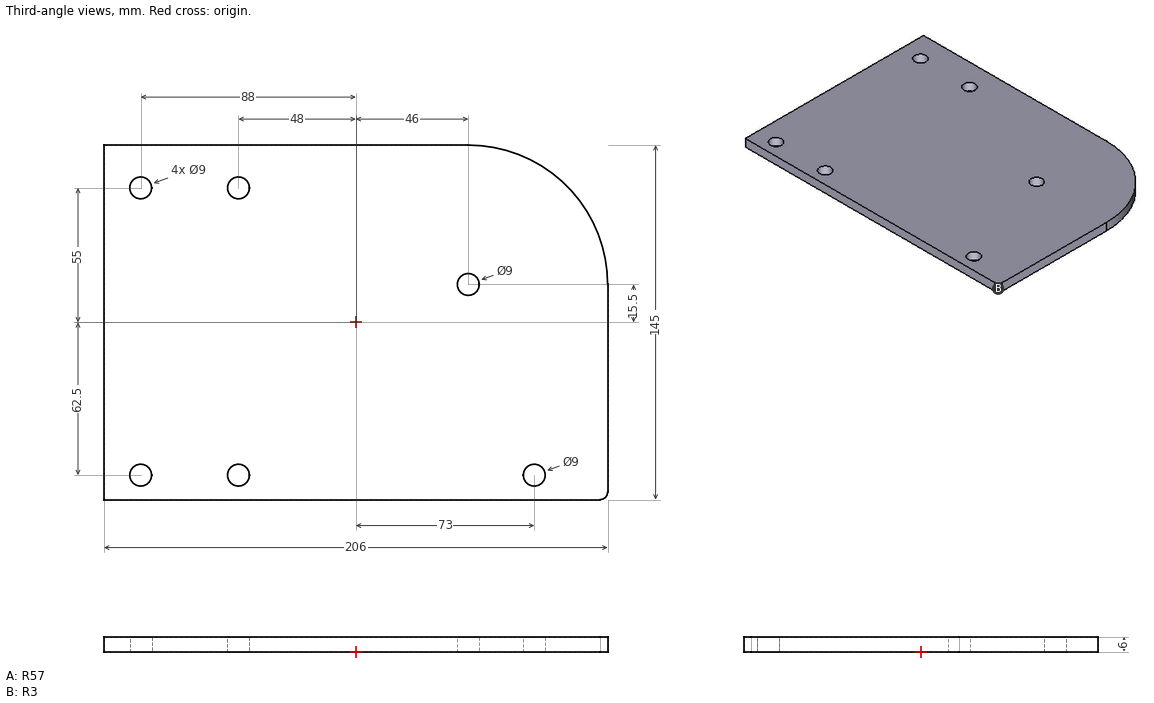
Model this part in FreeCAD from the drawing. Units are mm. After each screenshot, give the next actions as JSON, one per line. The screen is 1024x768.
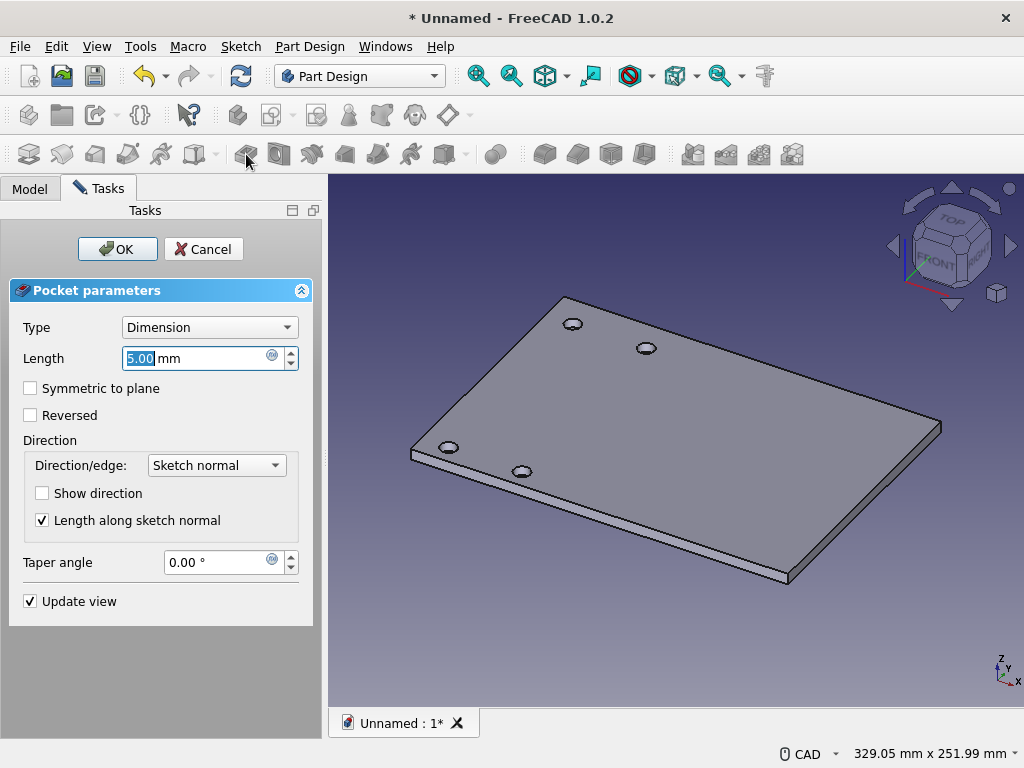
{"action": "left_click", "coordinate": [210, 328]}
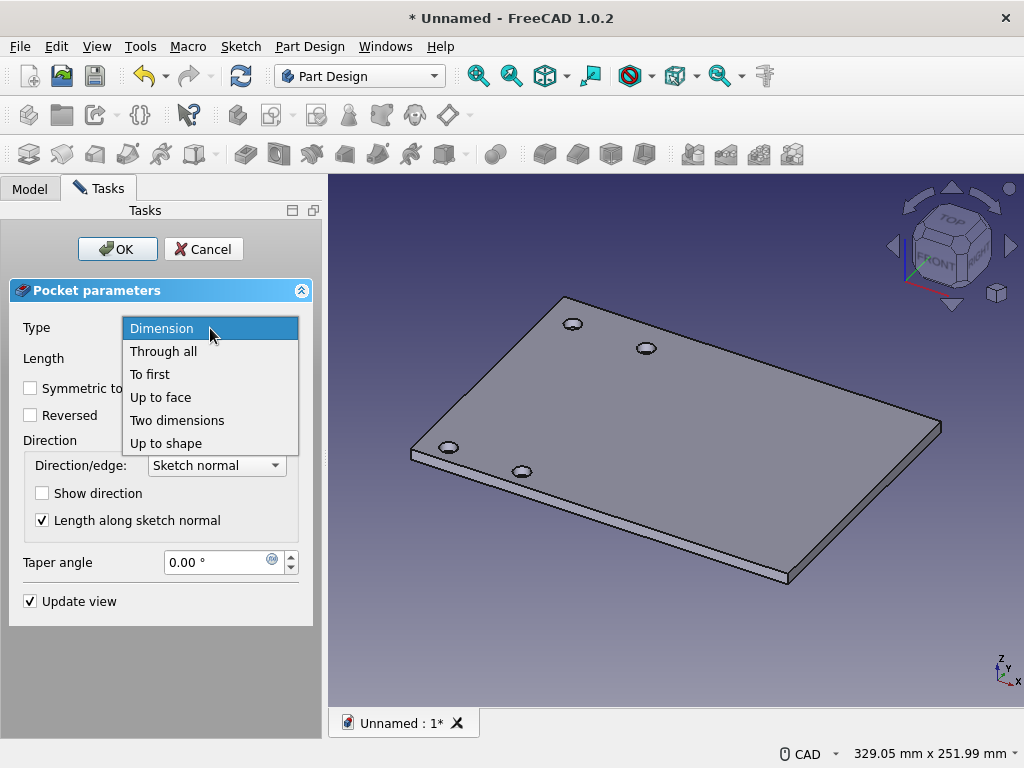
{"action": "left_click", "coordinate": [208, 352]}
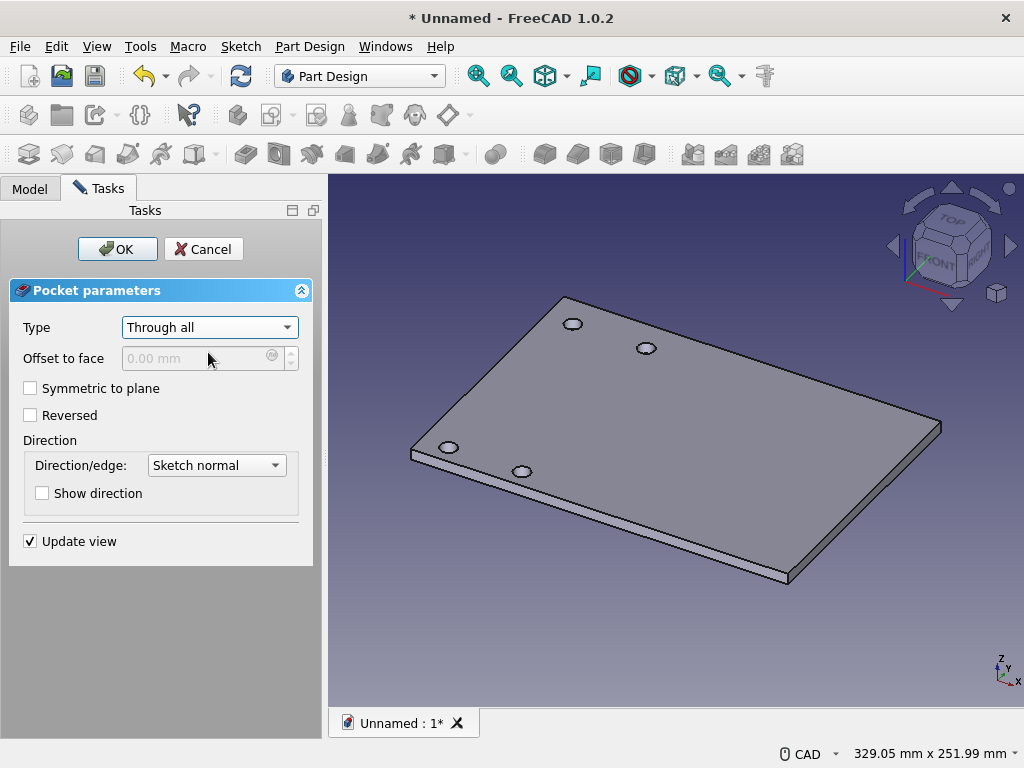
{"action": "left_click", "coordinate": [118, 249]}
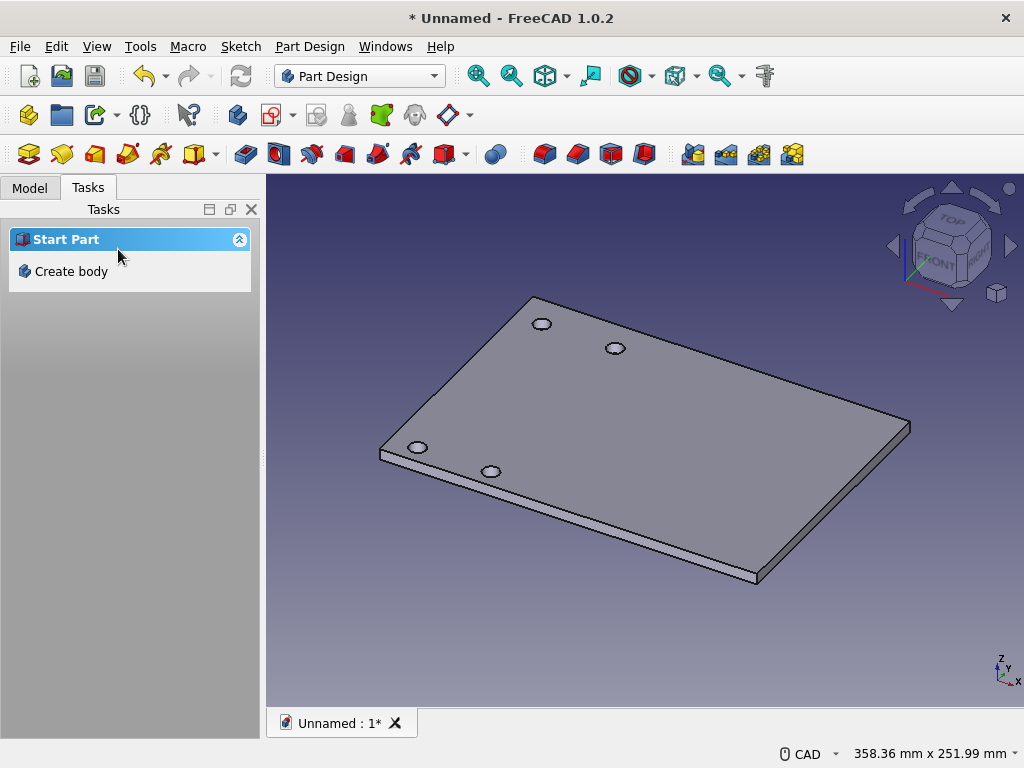
{"action": "left_click", "coordinate": [699, 452]}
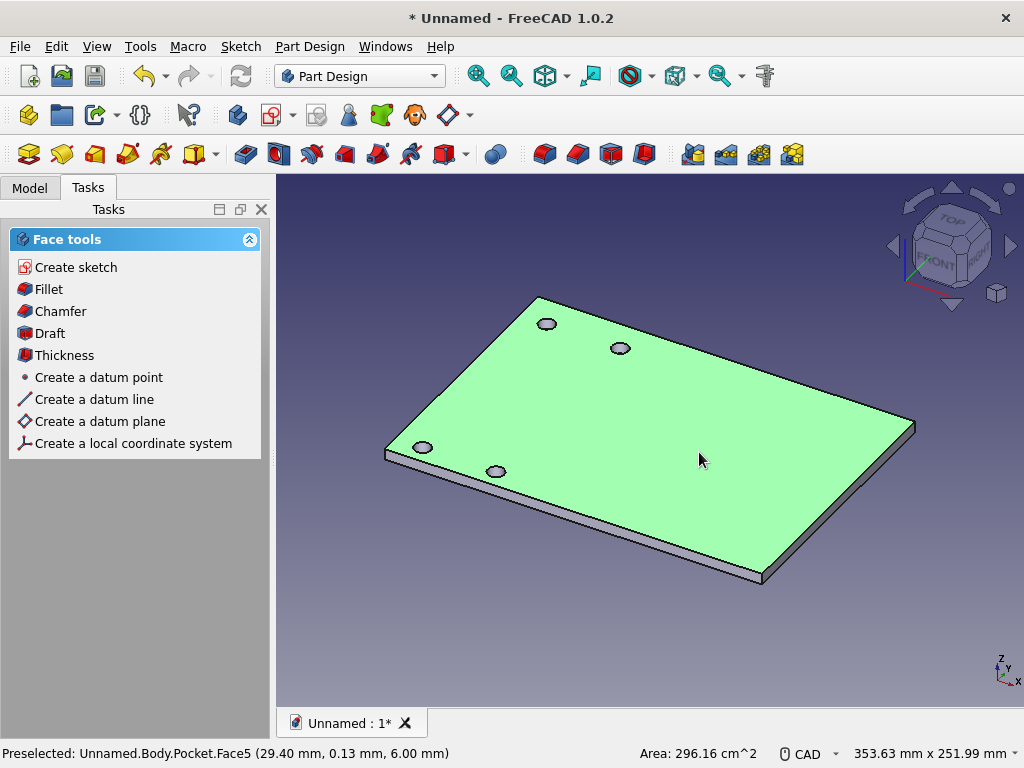
{"action": "left_click", "coordinate": [270, 116]}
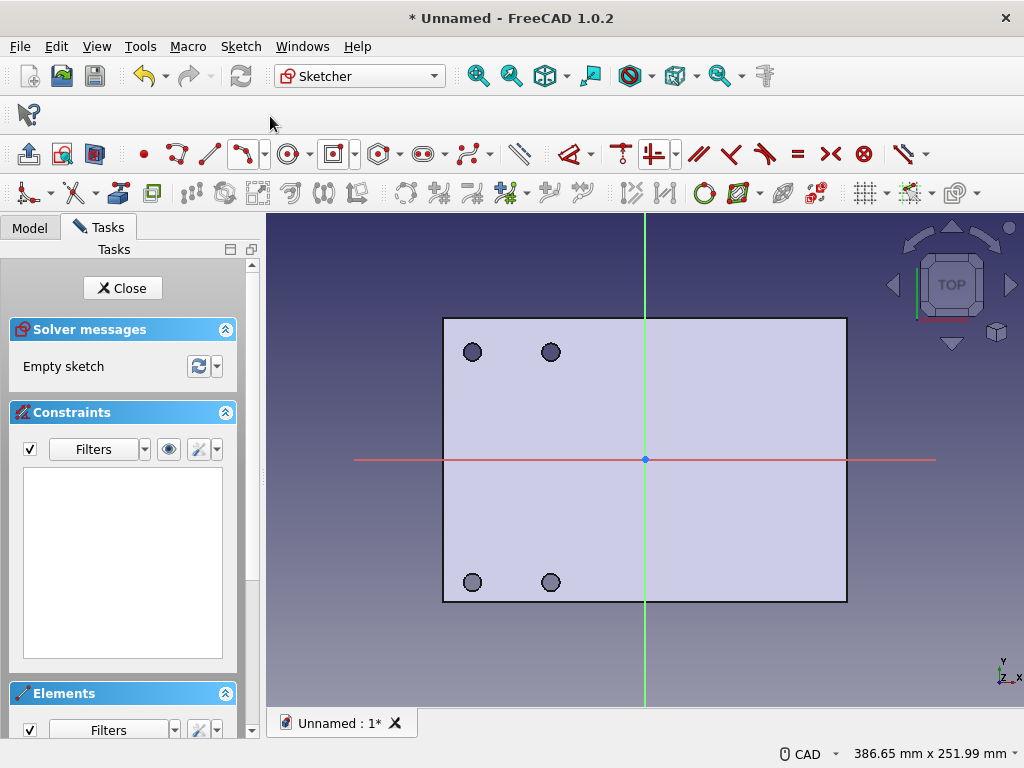
{"action": "scroll", "coordinate": [745, 428], "scroll_direction": "up", "scroll_amount": 14}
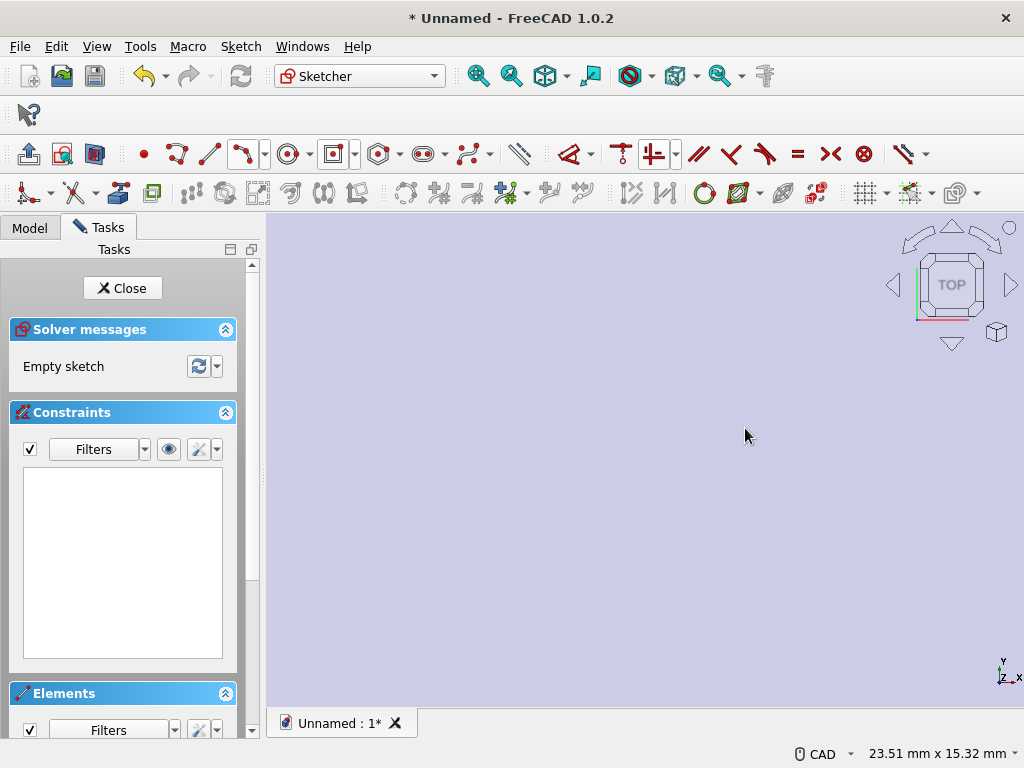
{"action": "key", "text": "g c"}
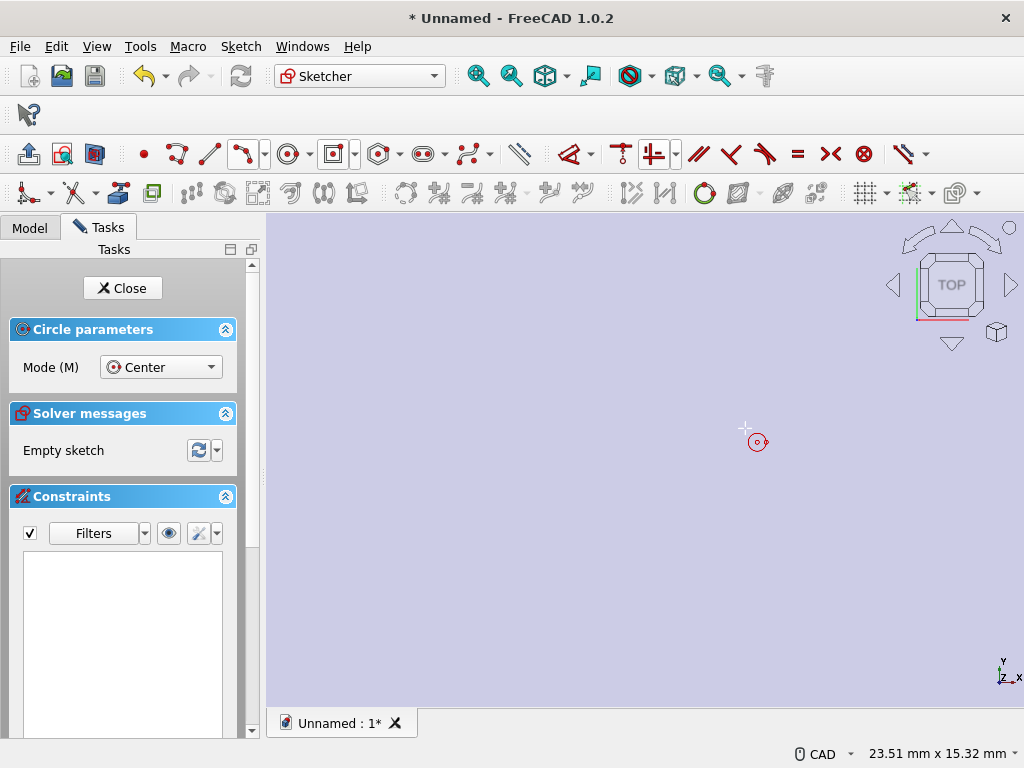
{"action": "left_click", "coordinate": [574, 448]}
{"action": "mouse_move", "coordinate": [676, 345]}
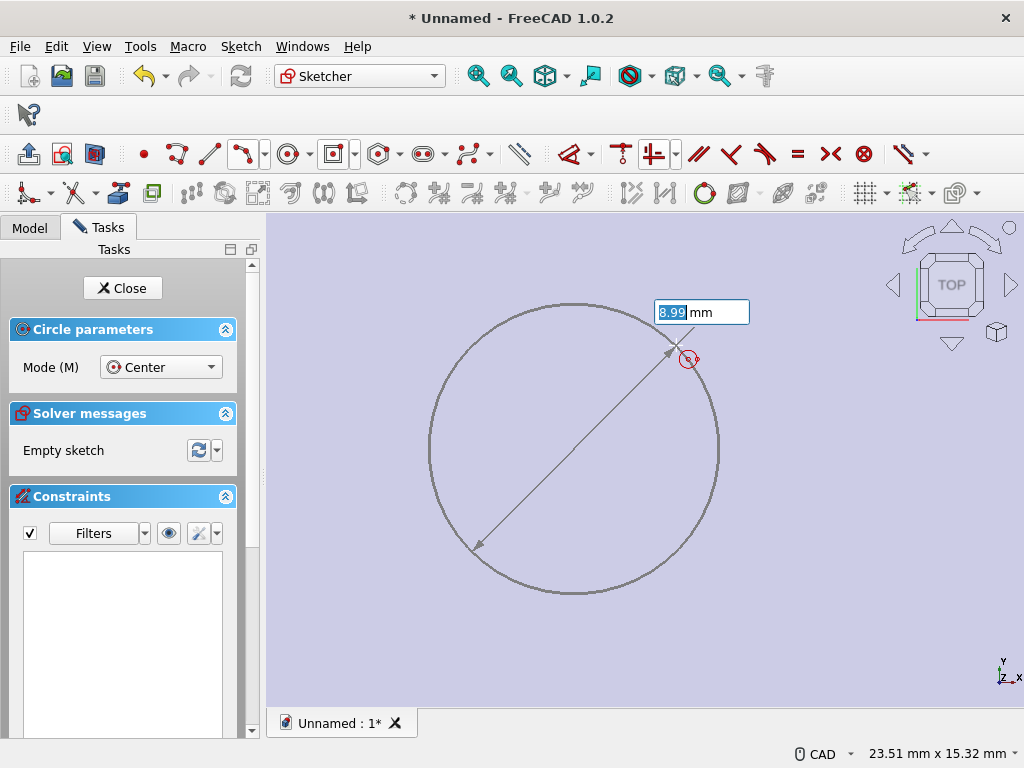
{"action": "type", "text": "9"}
{"action": "key", "text": "Return"}
{"action": "key", "text": "Escape"}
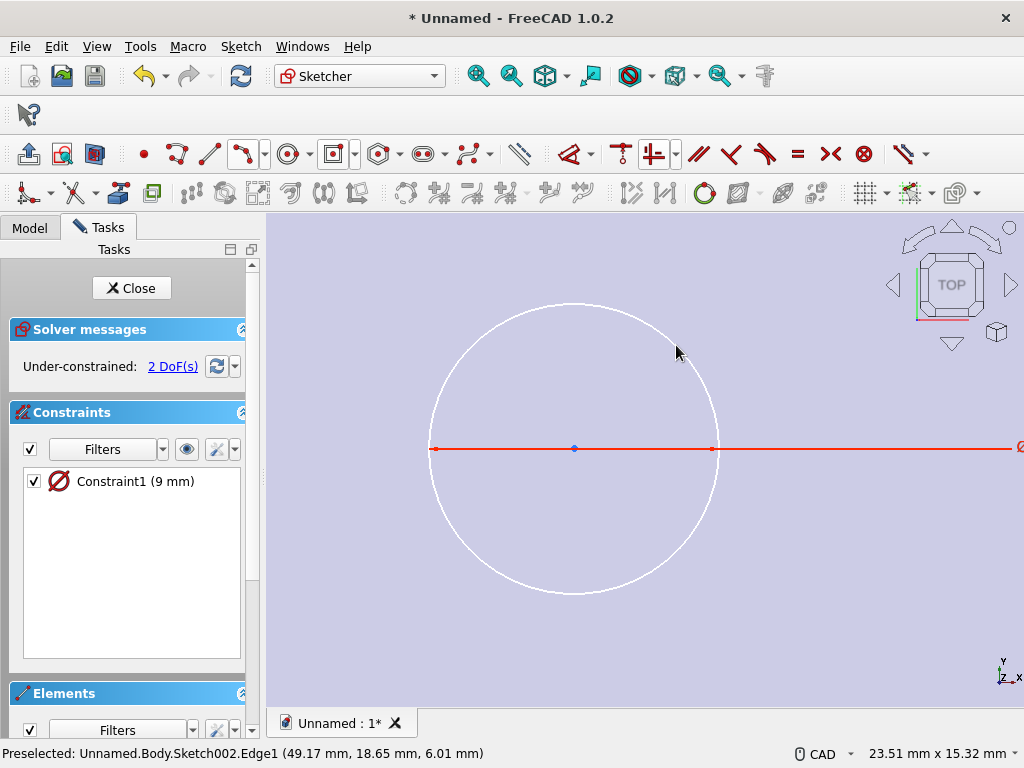
{"action": "left_click", "coordinate": [568, 154]}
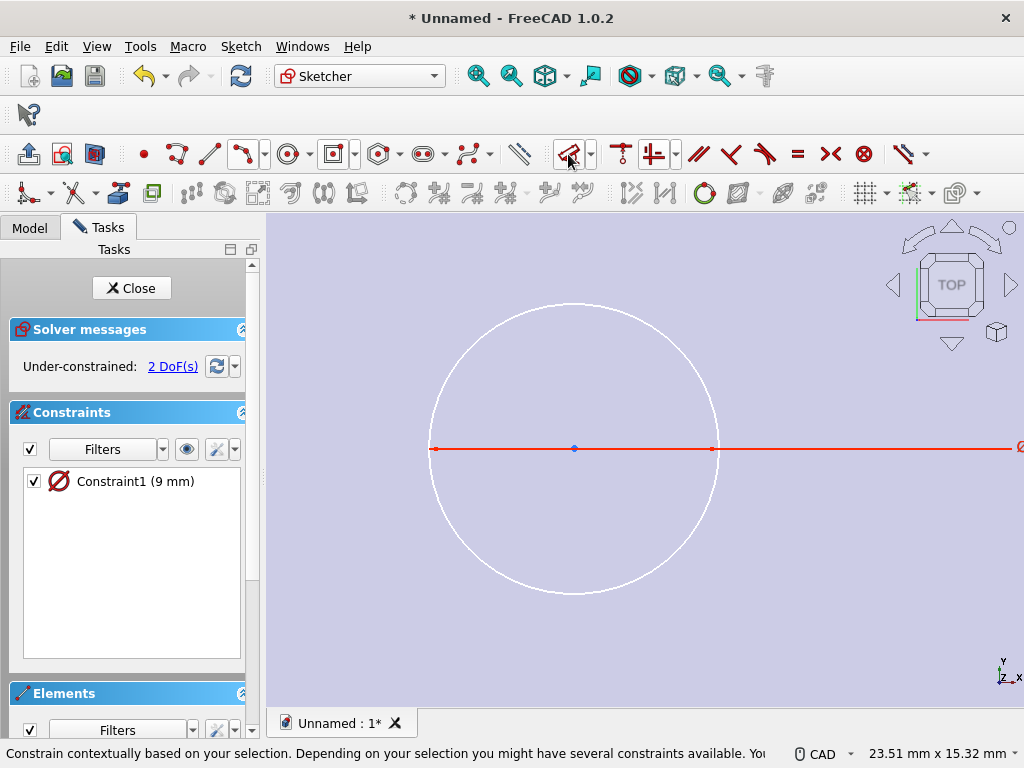
{"action": "left_click", "coordinate": [574, 449]}
{"action": "left_click", "coordinate": [370, 415]}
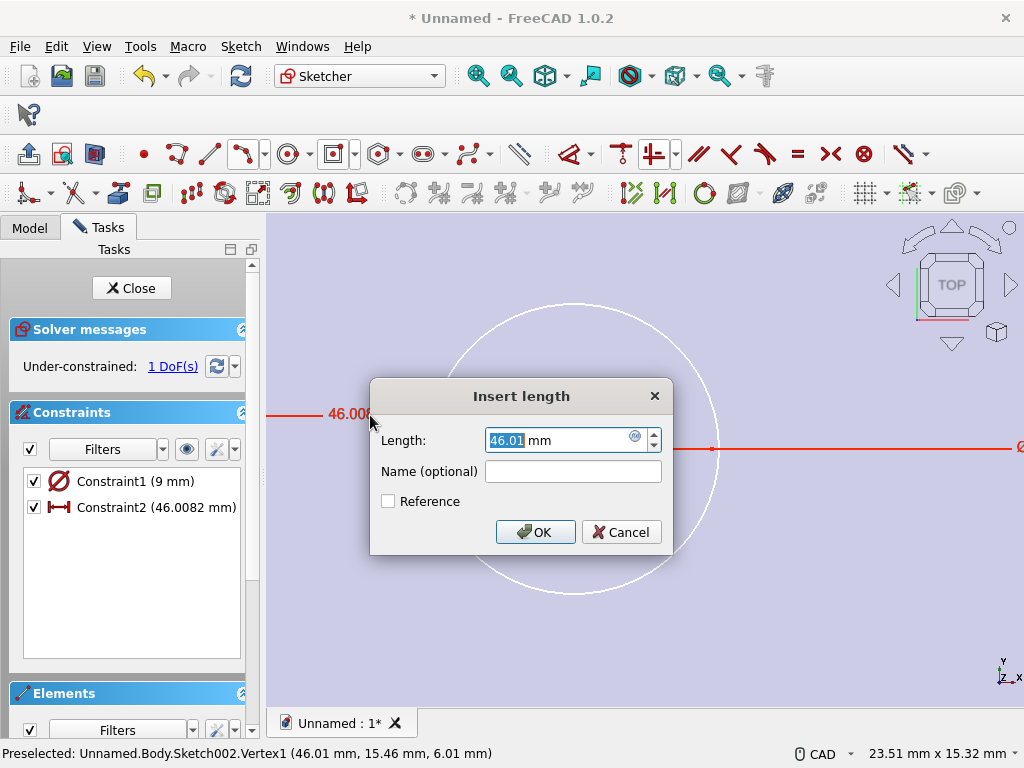
{"action": "type", "text": "46"}
{"action": "key", "text": "Return"}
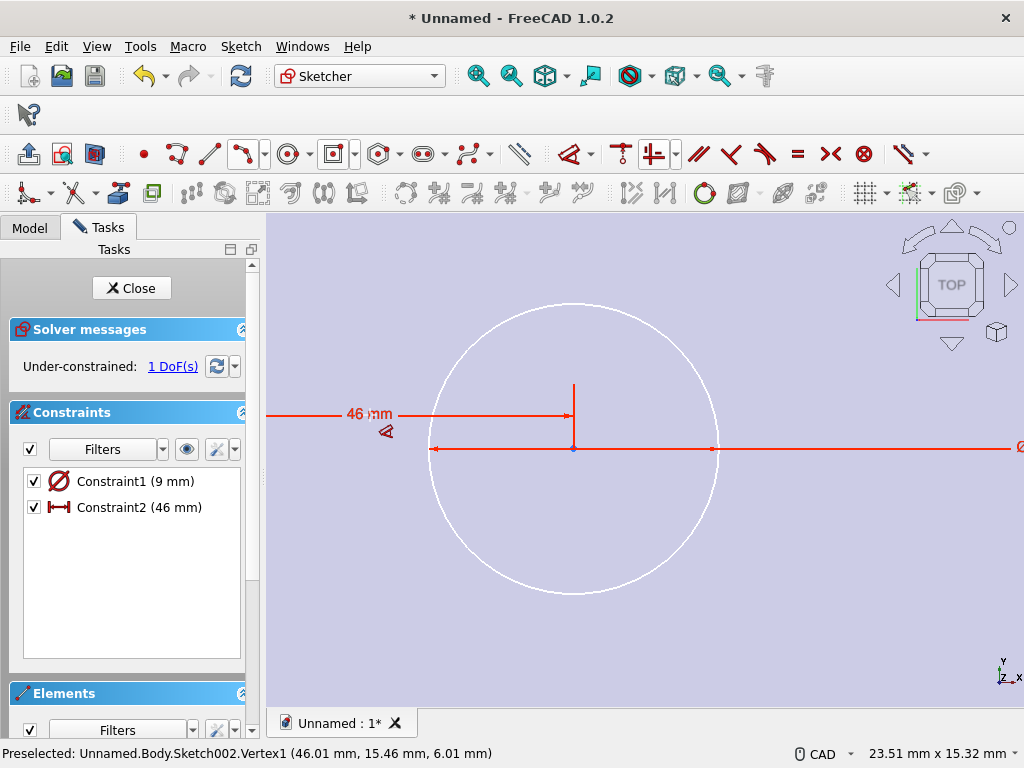
{"action": "left_click", "coordinate": [574, 449]}
{"action": "left_click", "coordinate": [608, 564]}